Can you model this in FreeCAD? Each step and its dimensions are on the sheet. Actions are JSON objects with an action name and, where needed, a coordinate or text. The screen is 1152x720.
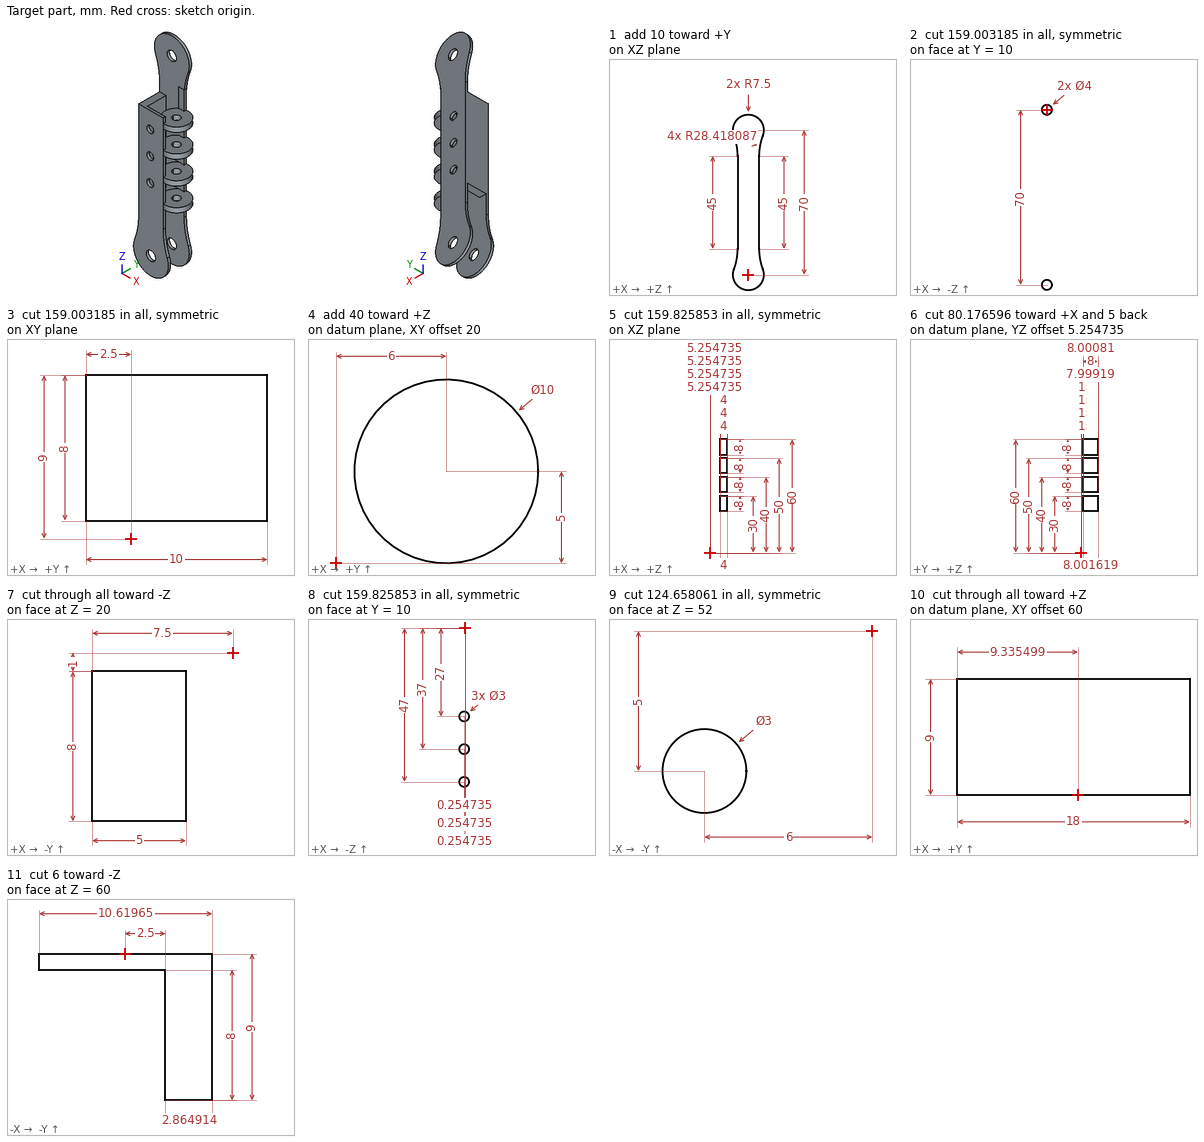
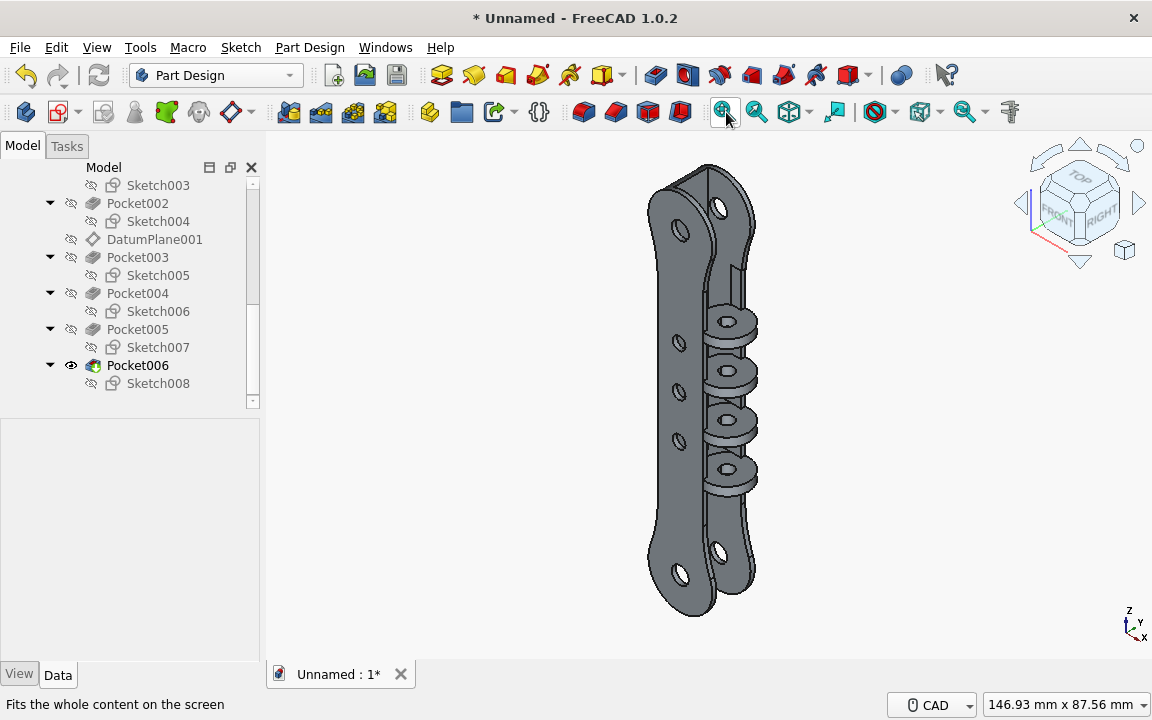
{"action": "scroll", "coordinate": [740, 269], "scroll_direction": "up", "scroll_amount": 15}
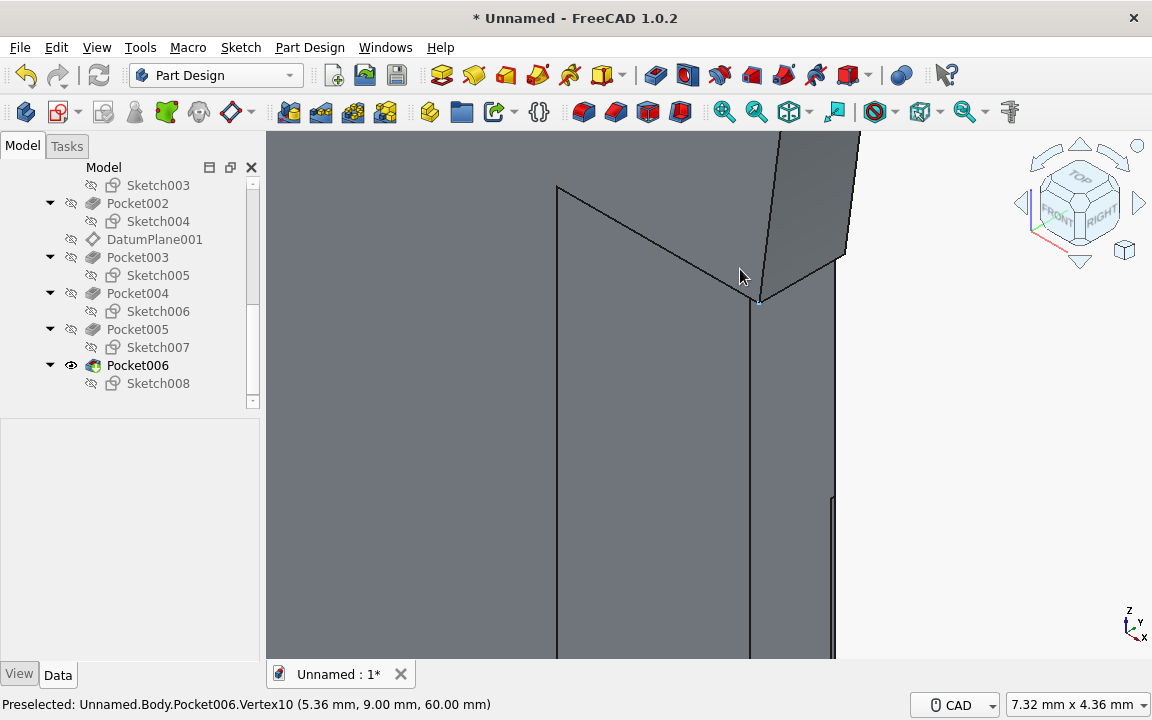
{"action": "scroll", "coordinate": [736, 289], "scroll_direction": "up", "scroll_amount": 15}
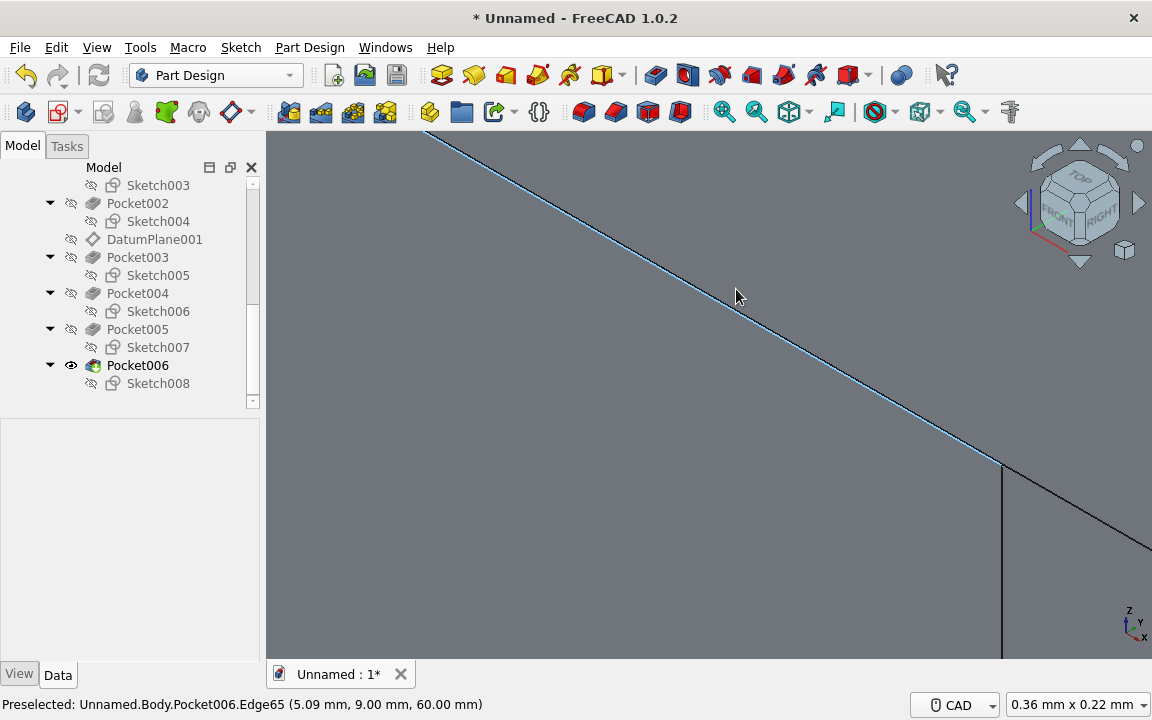
{"action": "left_click", "coordinate": [726, 112]}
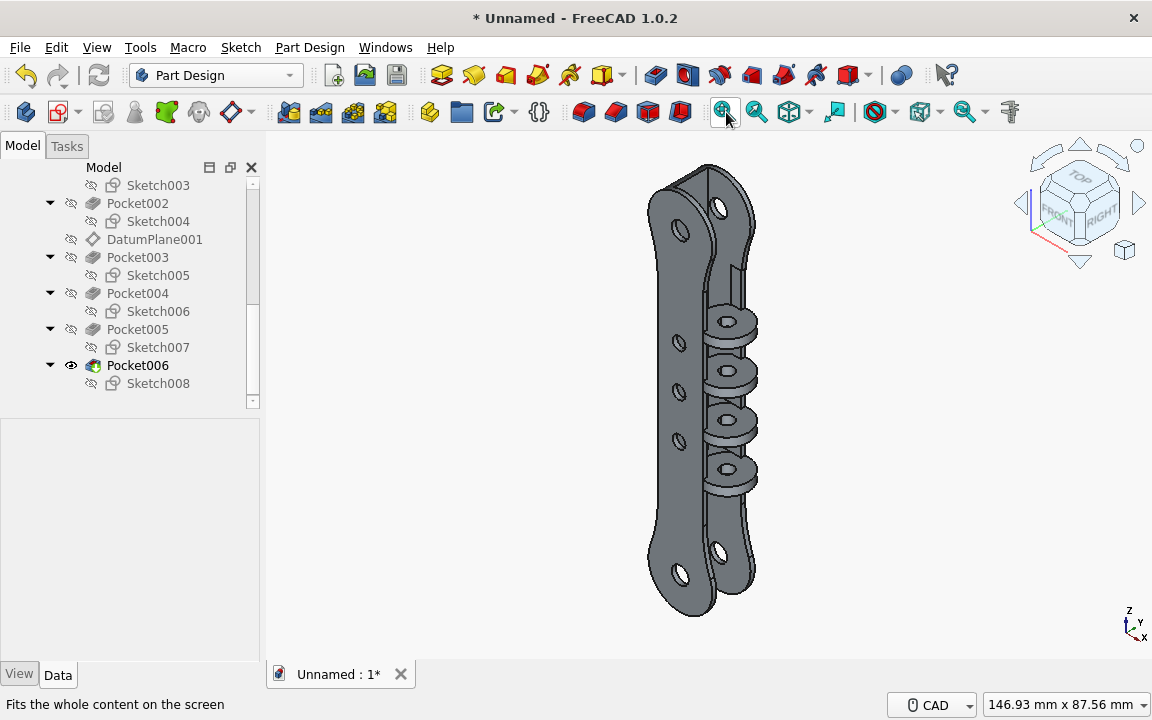
{"action": "key", "text": "4"}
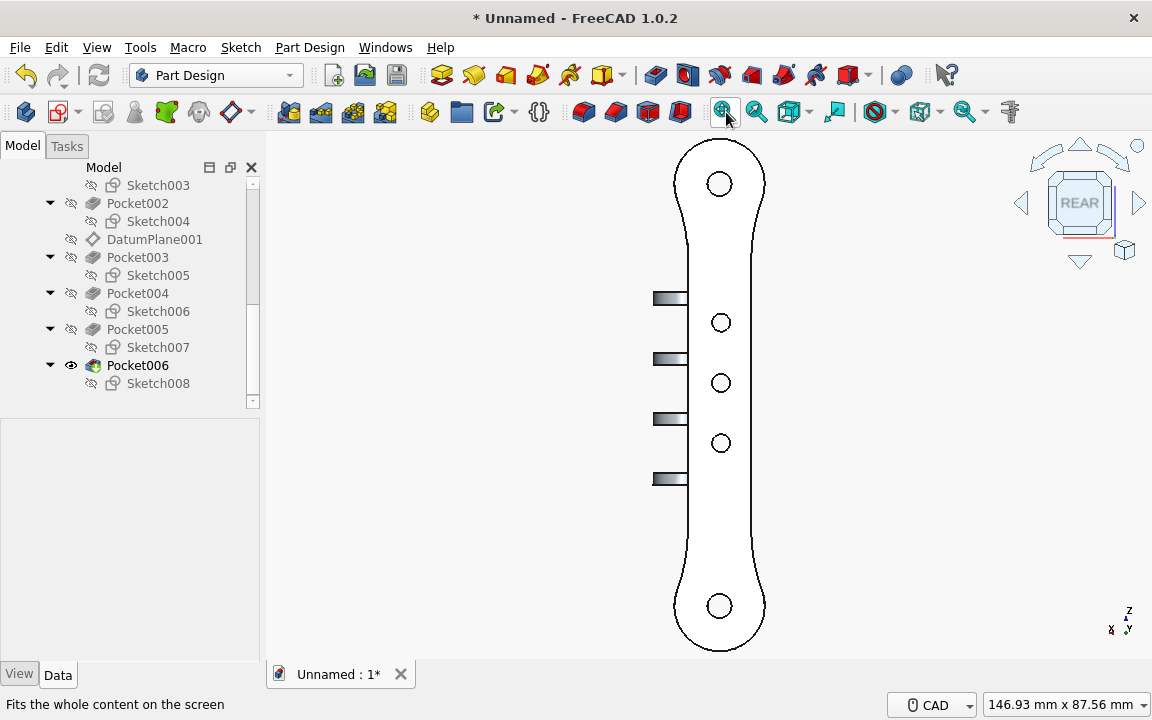
{"action": "scroll", "coordinate": [160, 289], "scroll_direction": "down", "scroll_amount": 3}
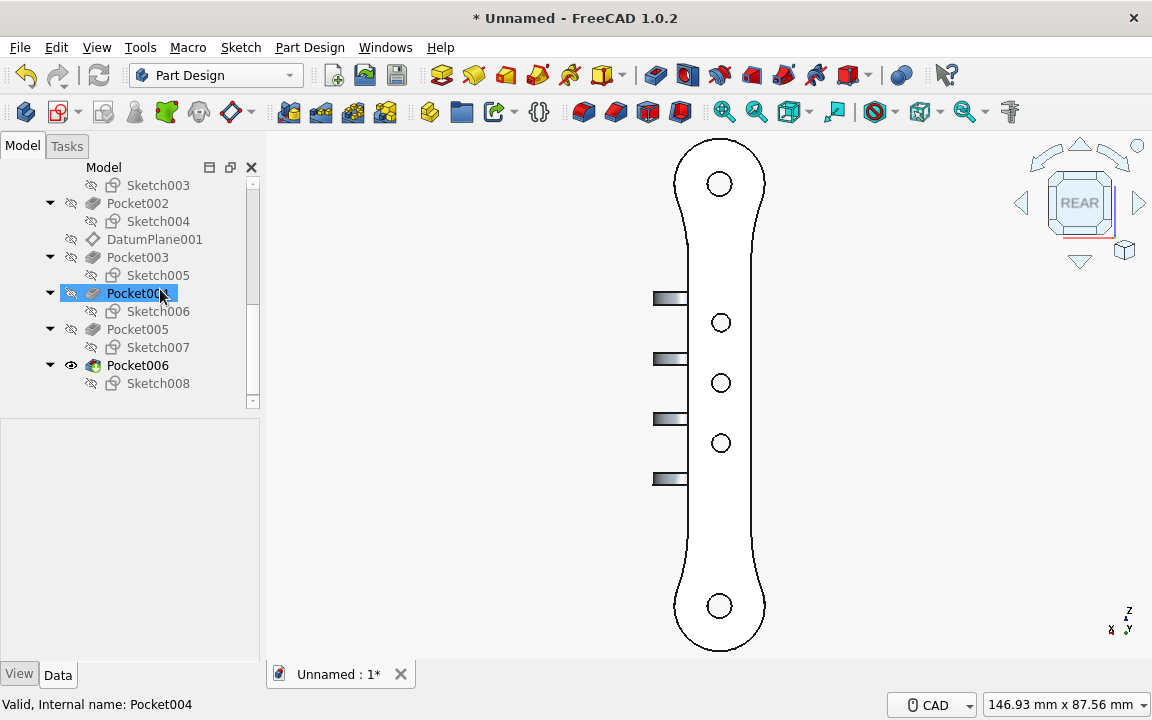
{"action": "scroll", "coordinate": [160, 289], "scroll_direction": "up", "scroll_amount": 15}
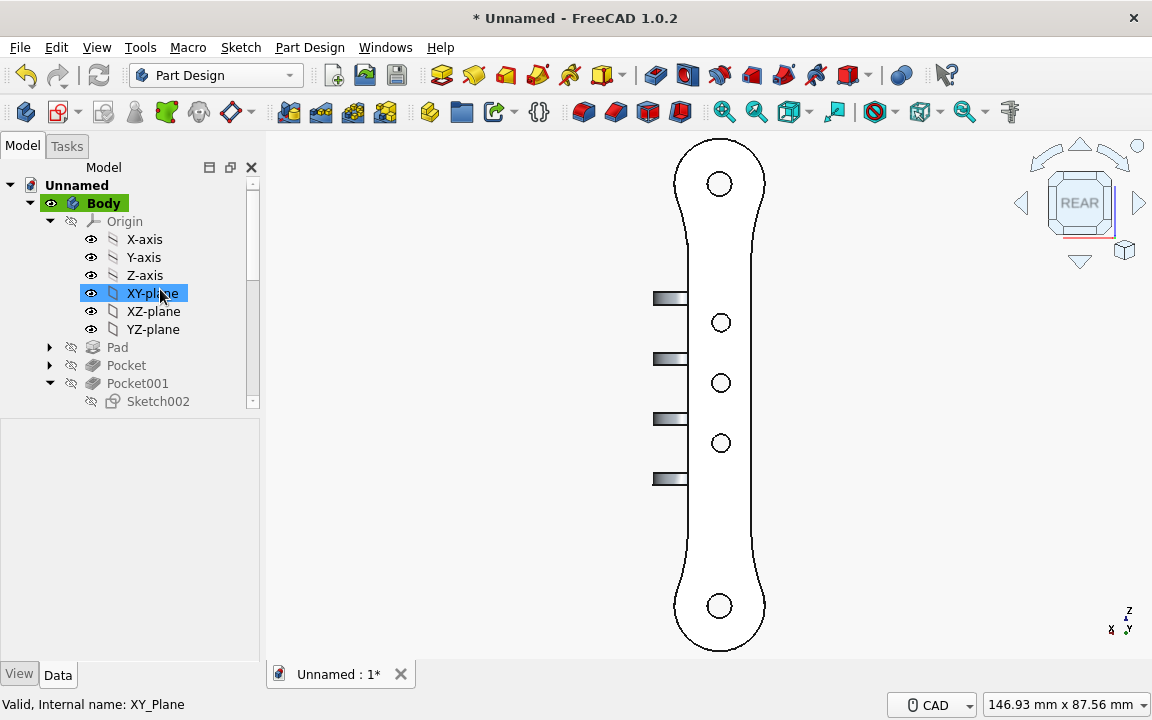
{"action": "left_click", "coordinate": [136, 293]}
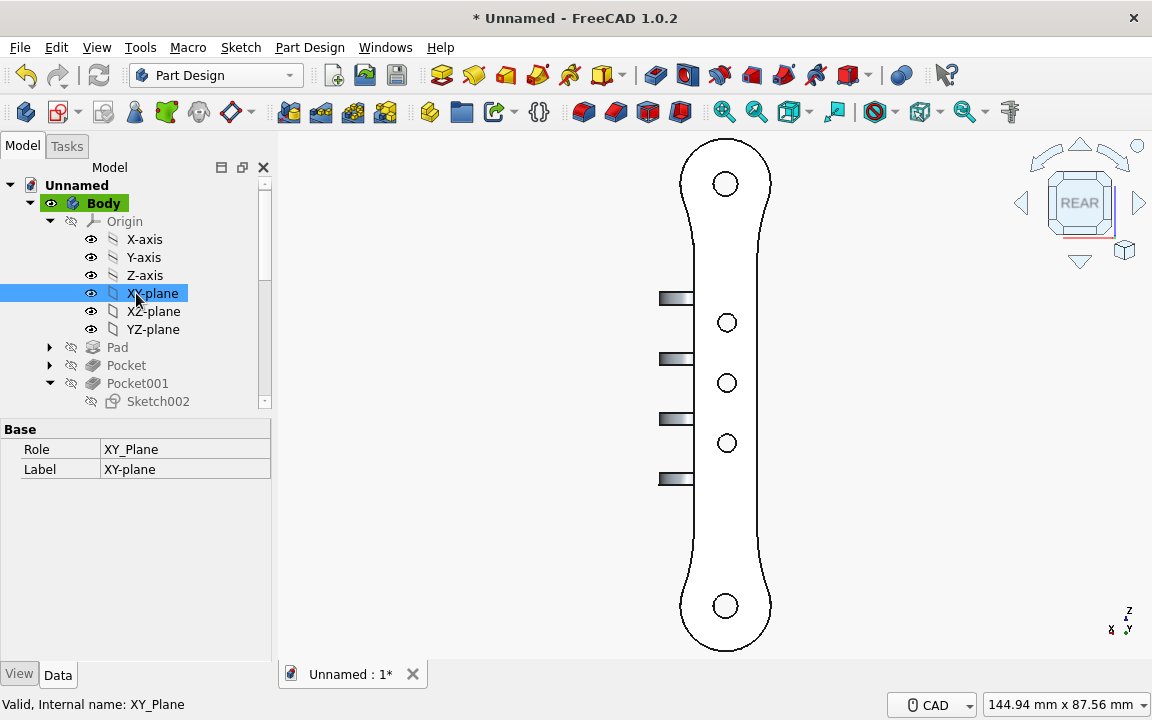
{"action": "left_click", "coordinate": [232, 112]}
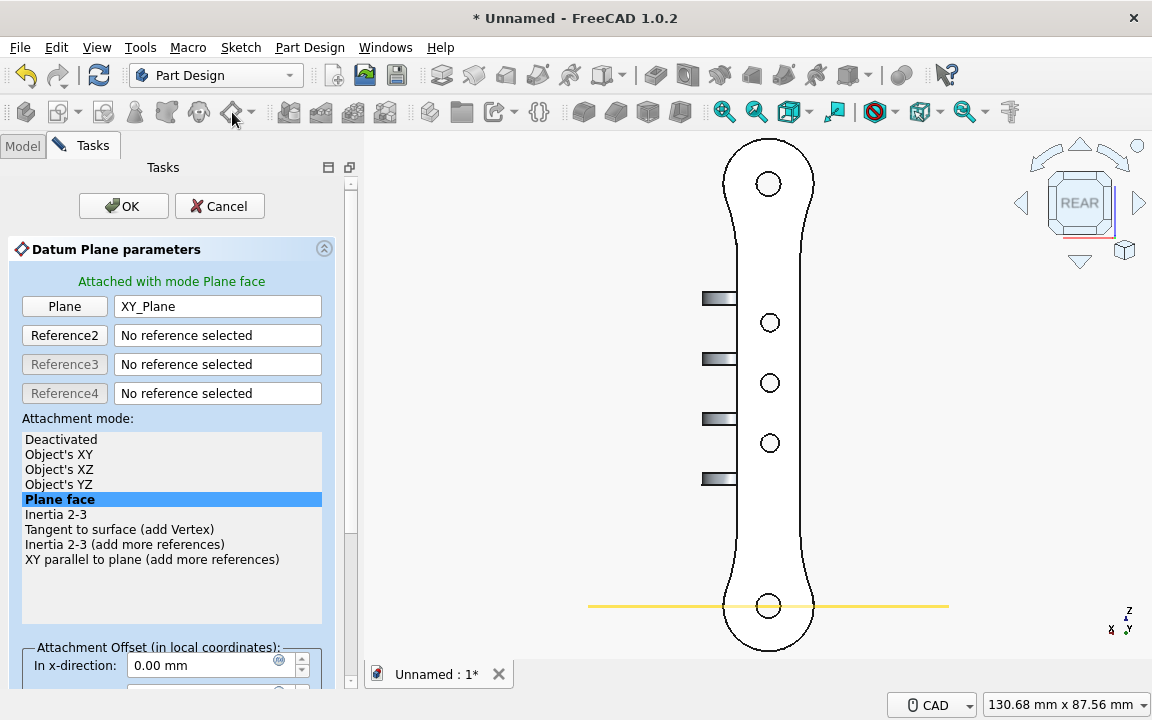
{"action": "scroll", "coordinate": [351, 432], "scroll_direction": "down", "scroll_amount": 2}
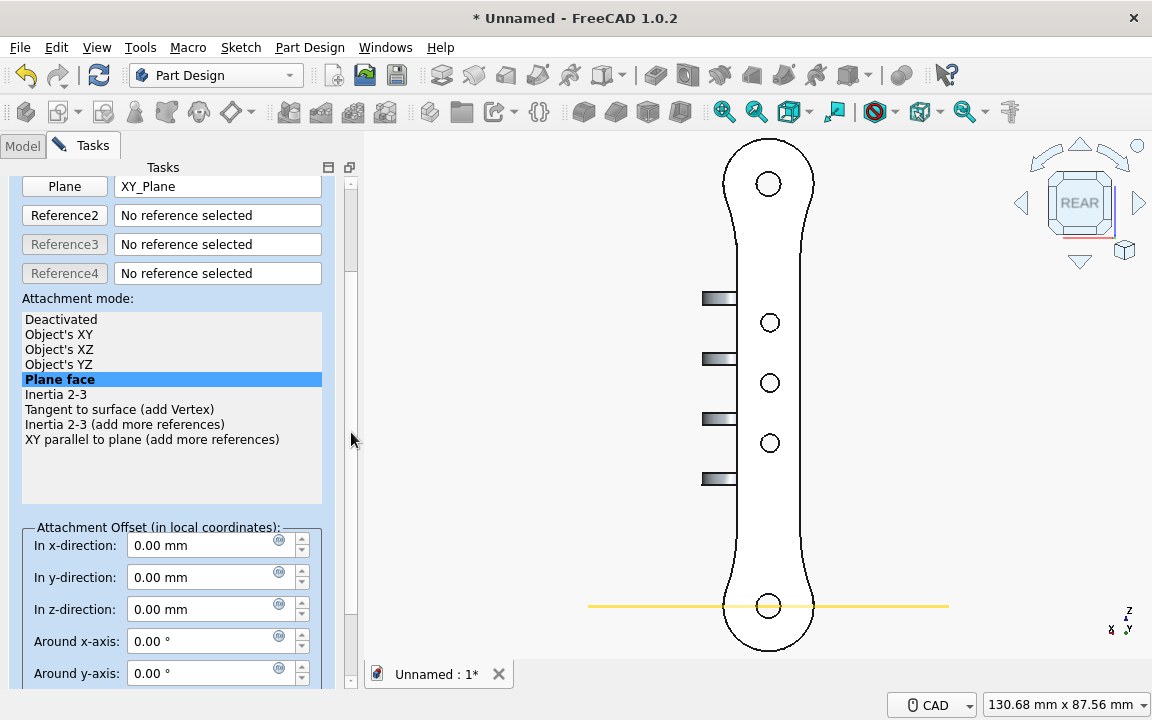
{"action": "triple_click", "coordinate": [210, 609]}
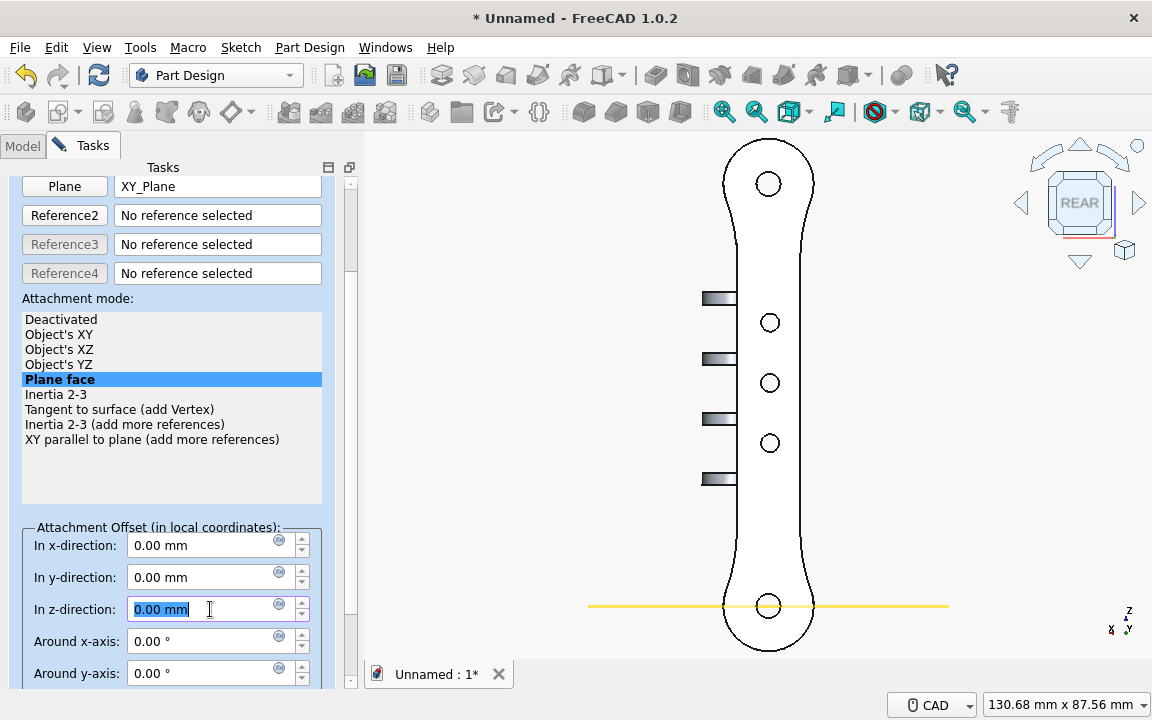
{"action": "type", "text": "60"}
{"action": "key", "text": "Tab"}